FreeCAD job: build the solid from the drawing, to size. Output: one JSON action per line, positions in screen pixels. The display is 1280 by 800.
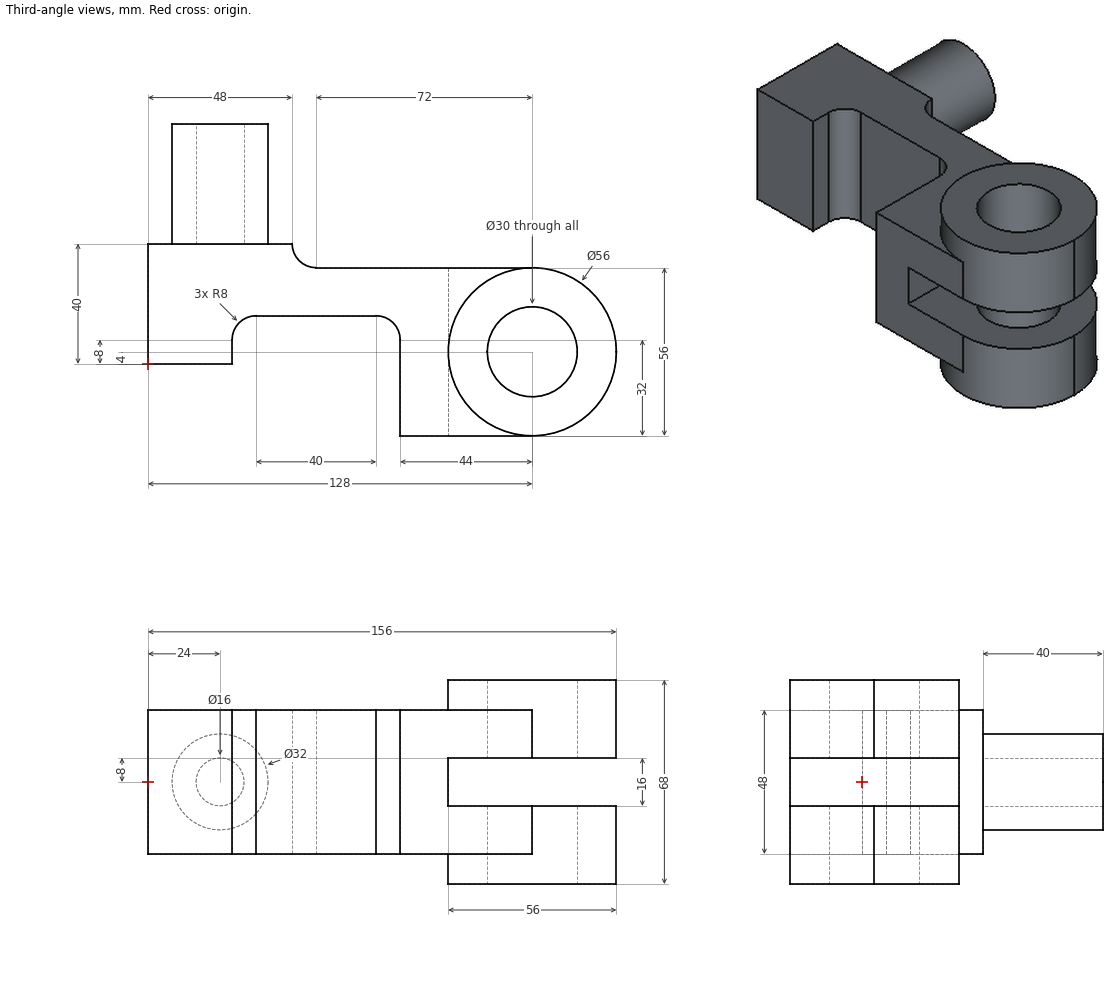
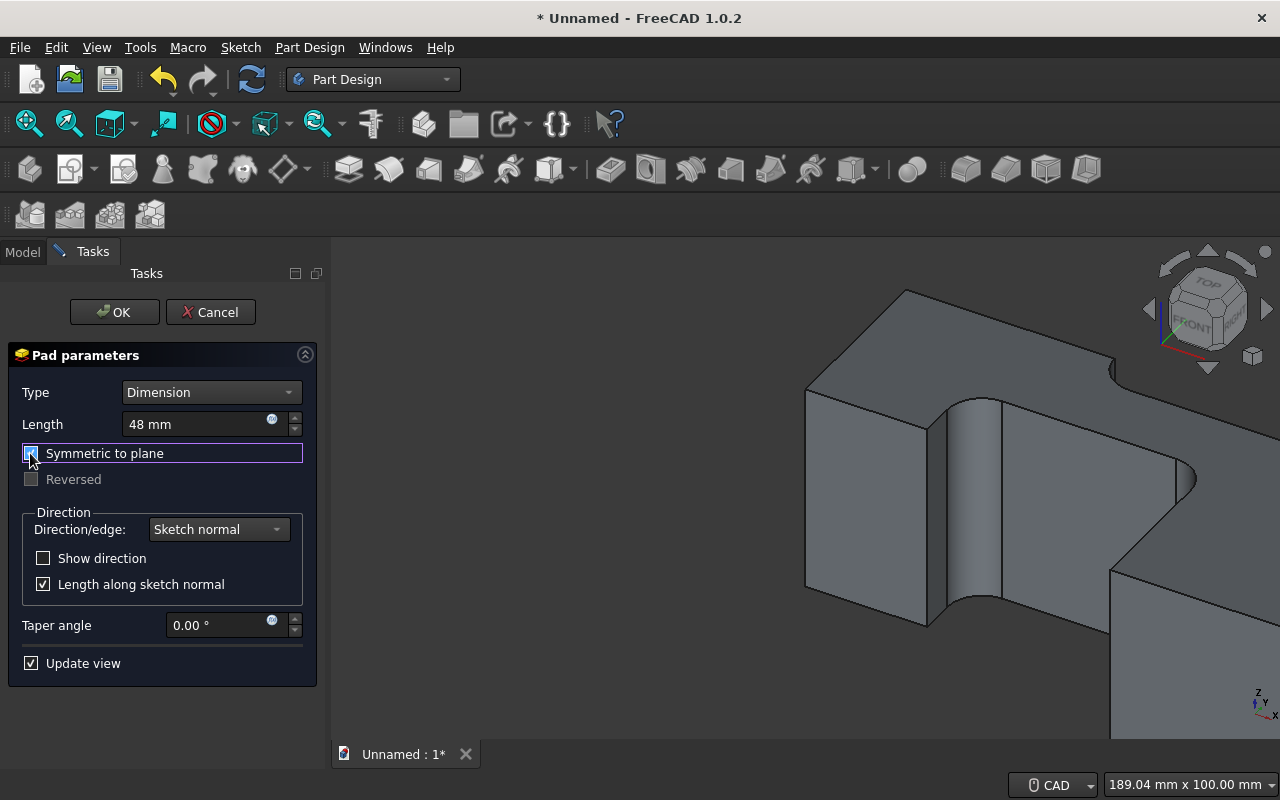
{"action": "left_click", "coordinate": [115, 312]}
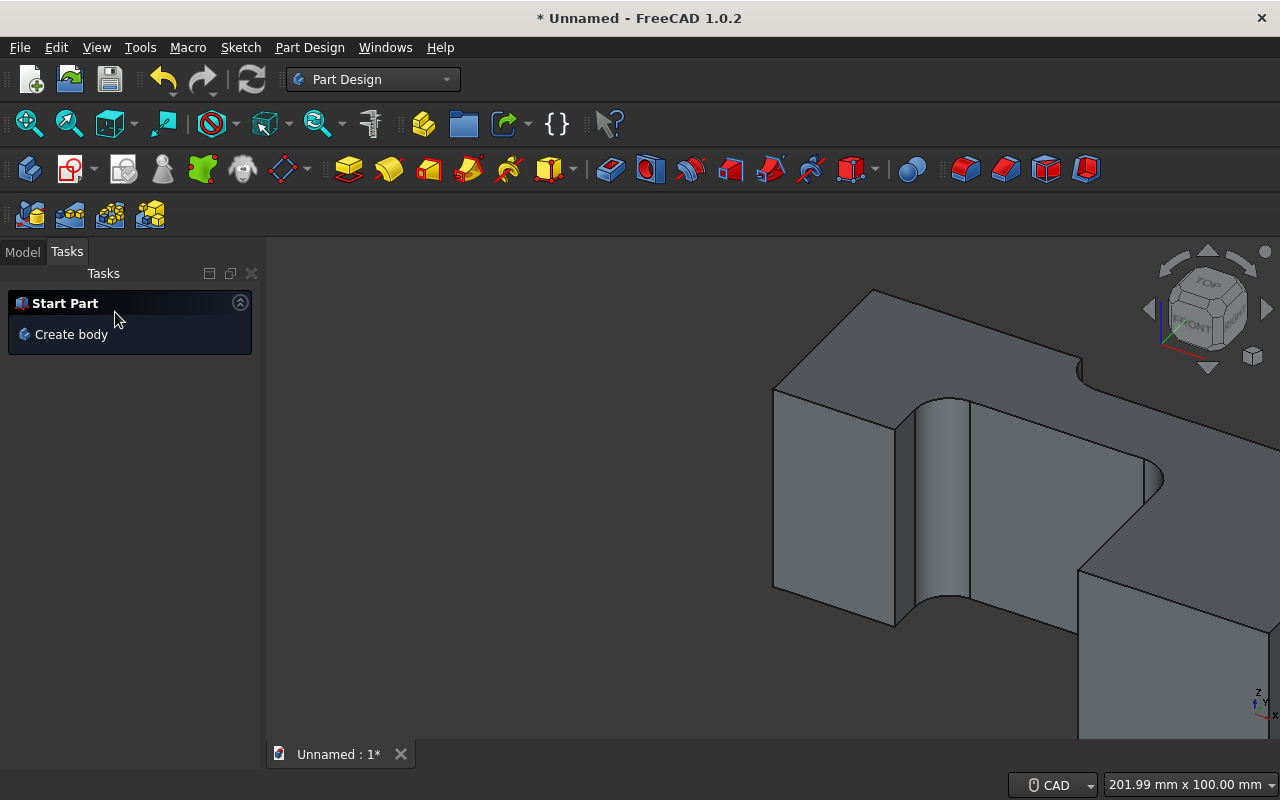
{"action": "left_click", "coordinate": [30, 124]}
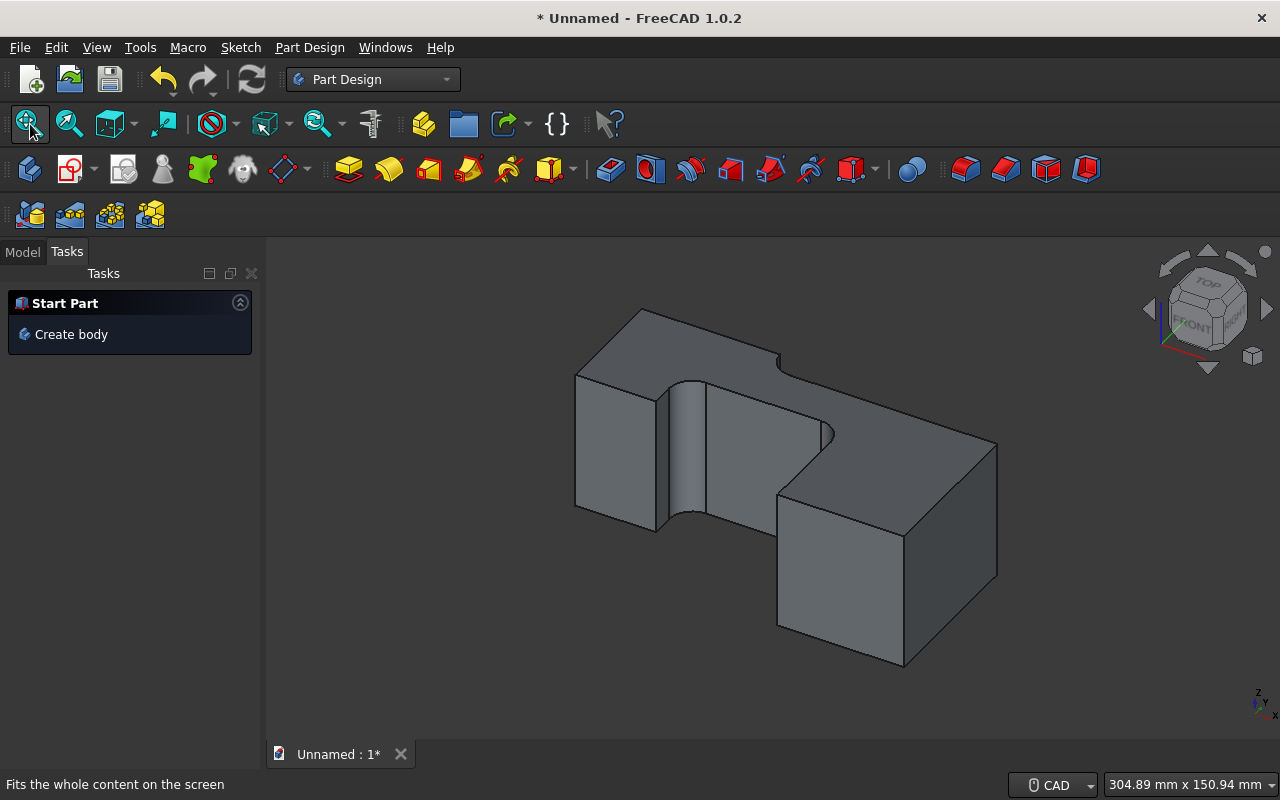
{"action": "key", "text": "4"}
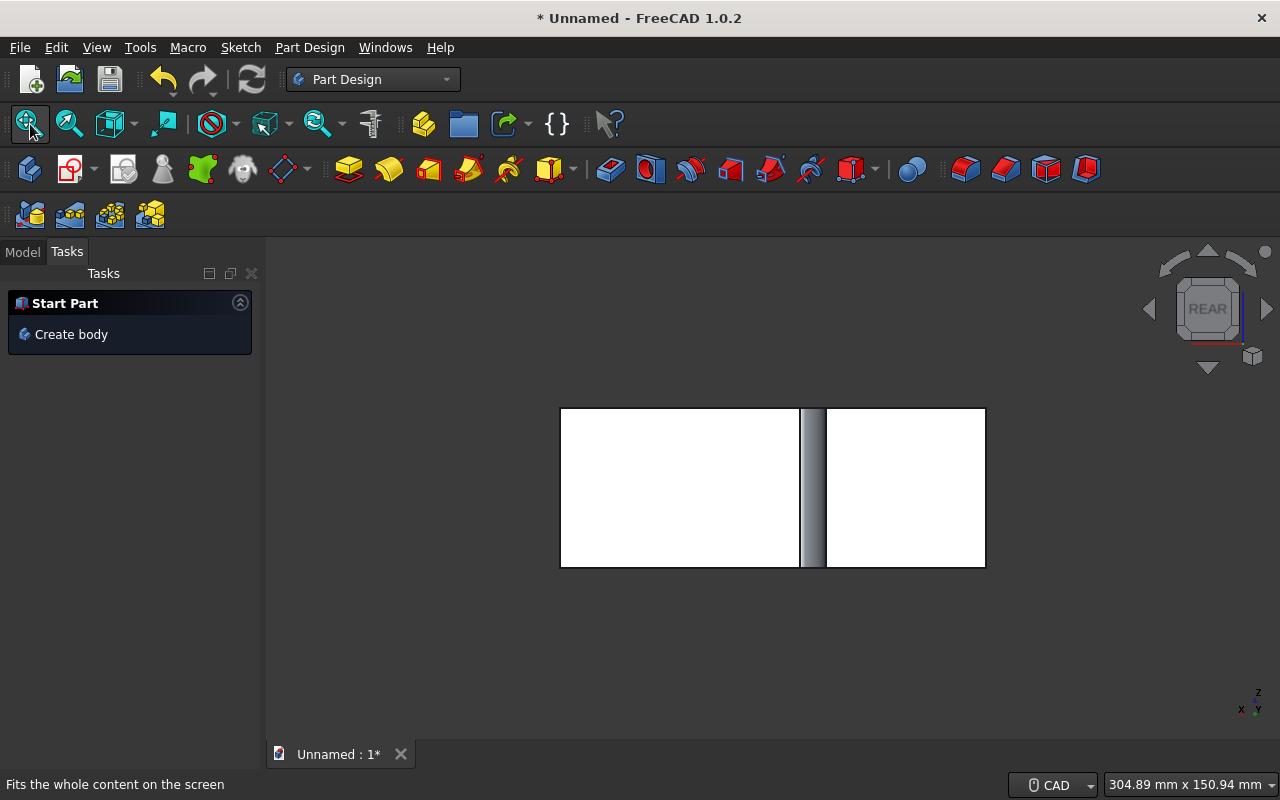
{"action": "left_click", "coordinate": [30, 124]}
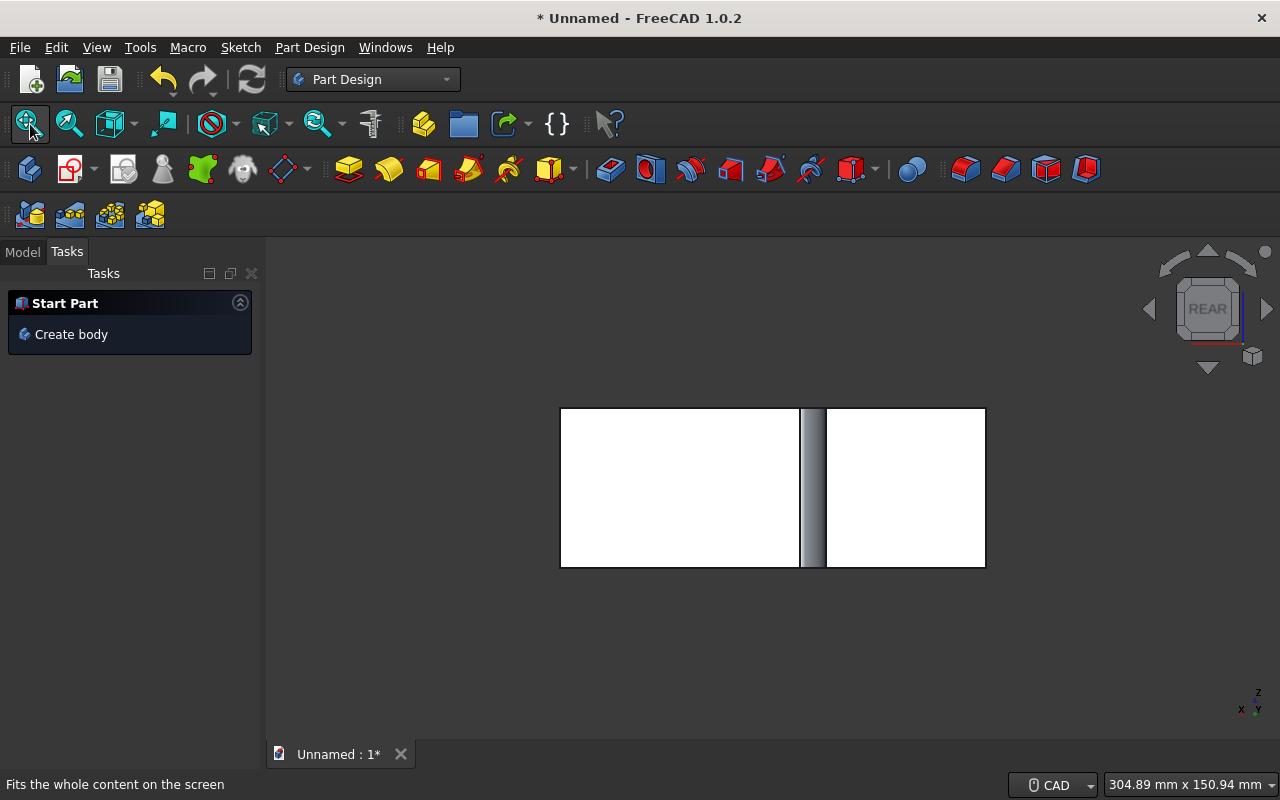
{"action": "left_click", "coordinate": [906, 487]}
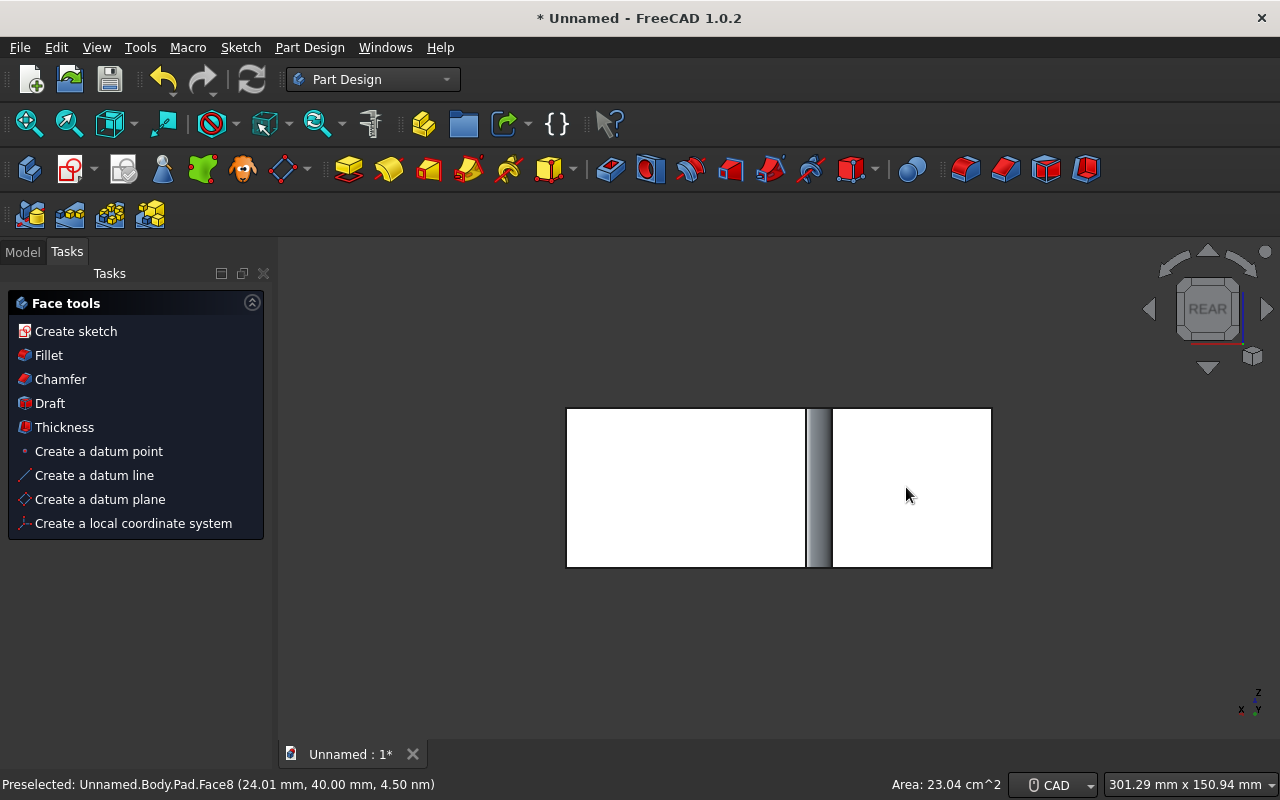
{"action": "left_click", "coordinate": [70, 170]}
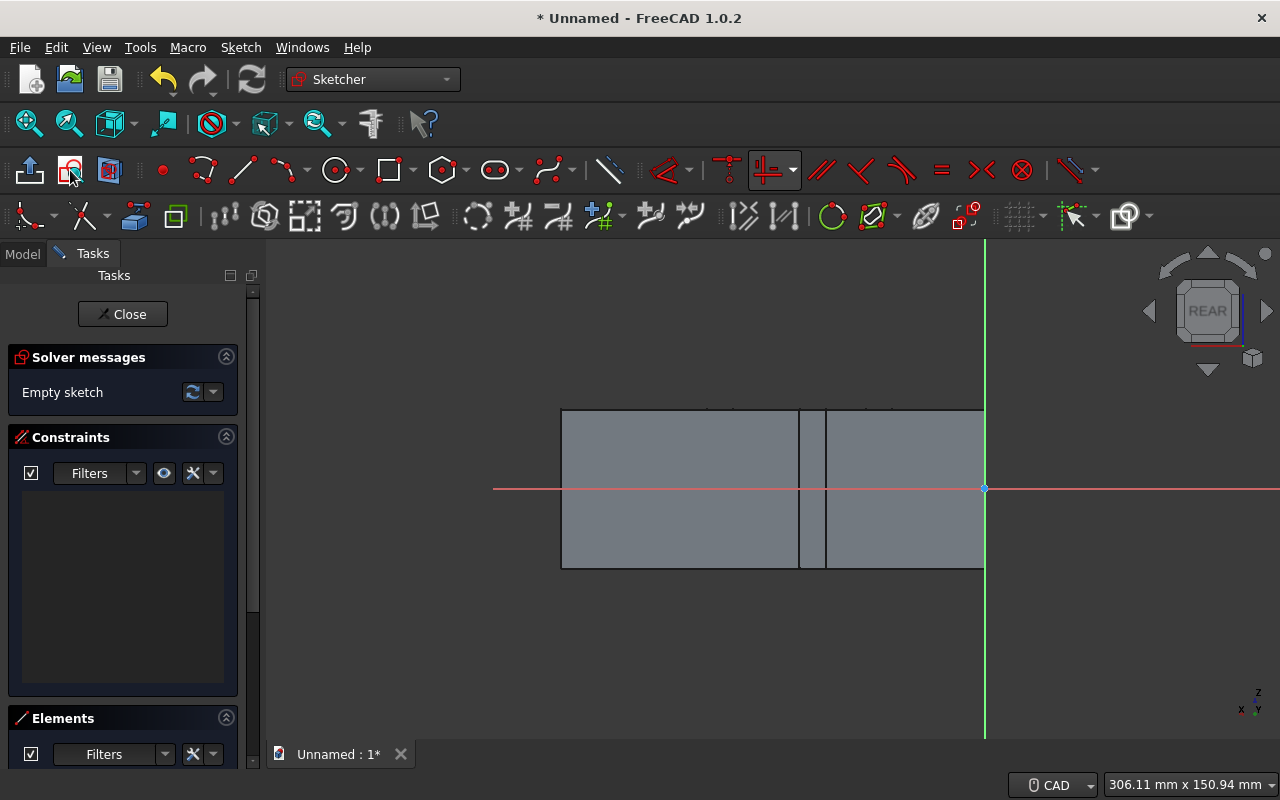
{"action": "scroll", "coordinate": [1043, 489], "scroll_direction": "up", "scroll_amount": 5}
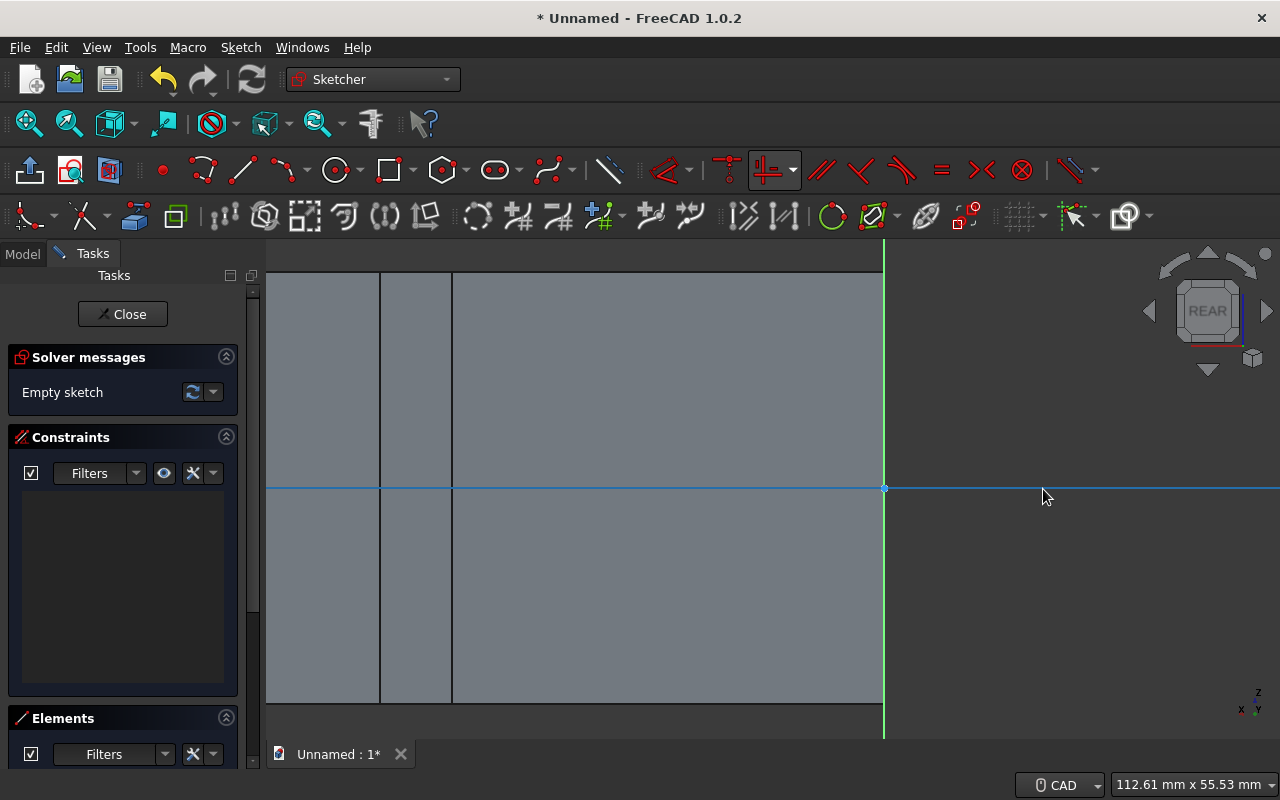
{"action": "key", "text": "g c"}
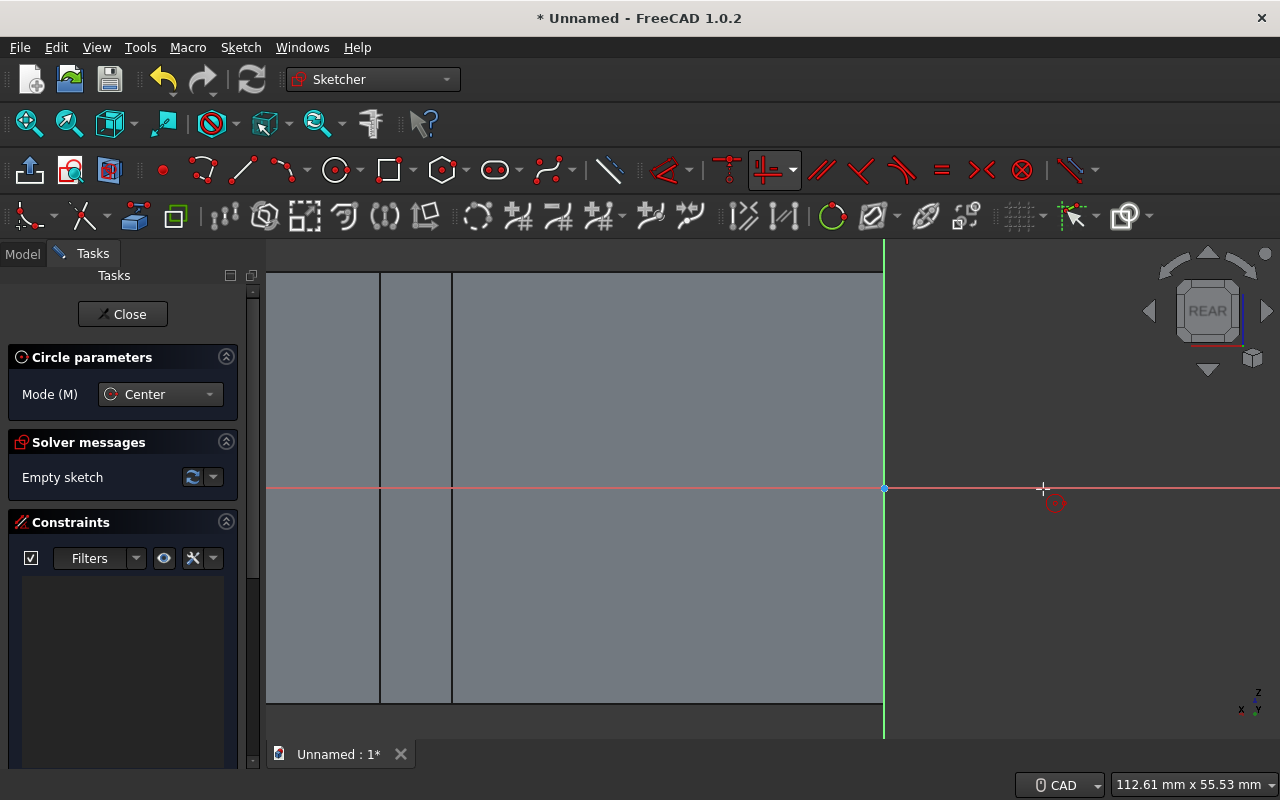
{"action": "left_click", "coordinate": [668, 488]}
{"action": "mouse_move", "coordinate": [770, 386]}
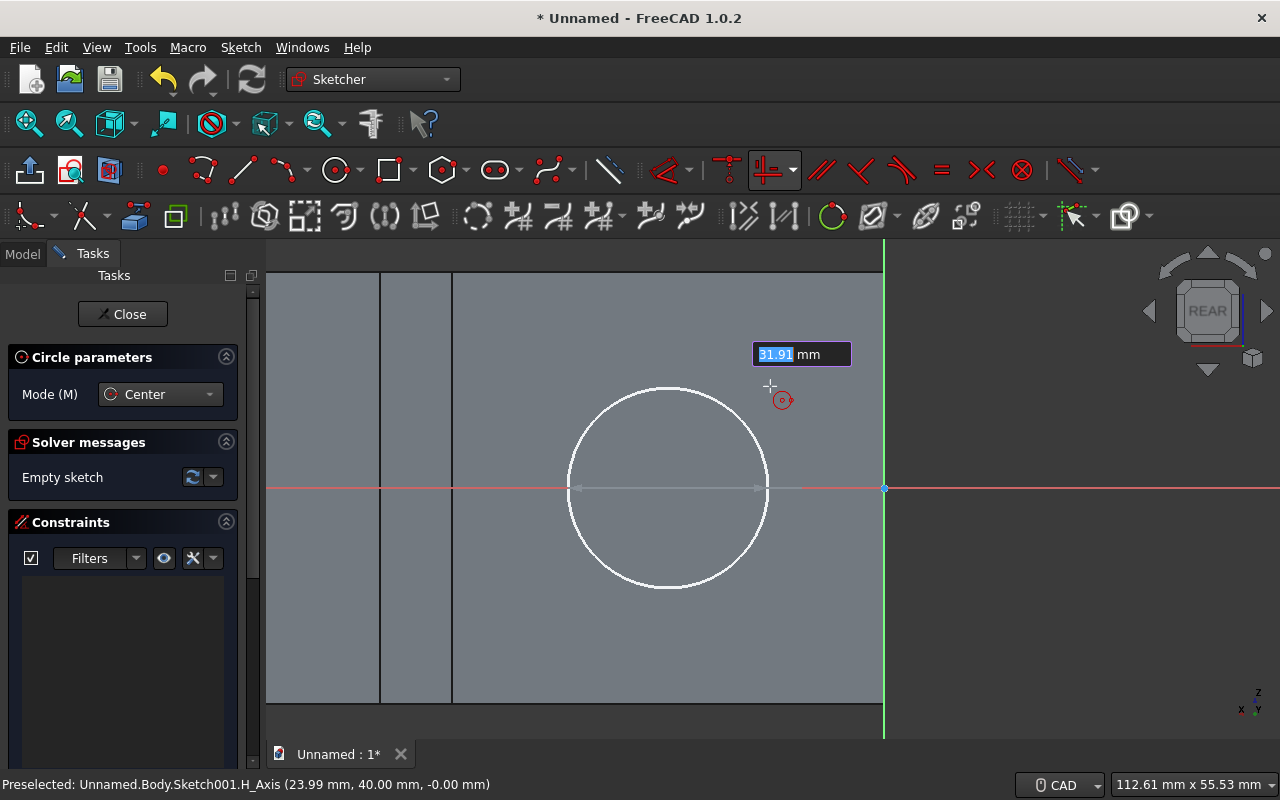
{"action": "type", "text": "32"}
{"action": "key", "text": "Return"}